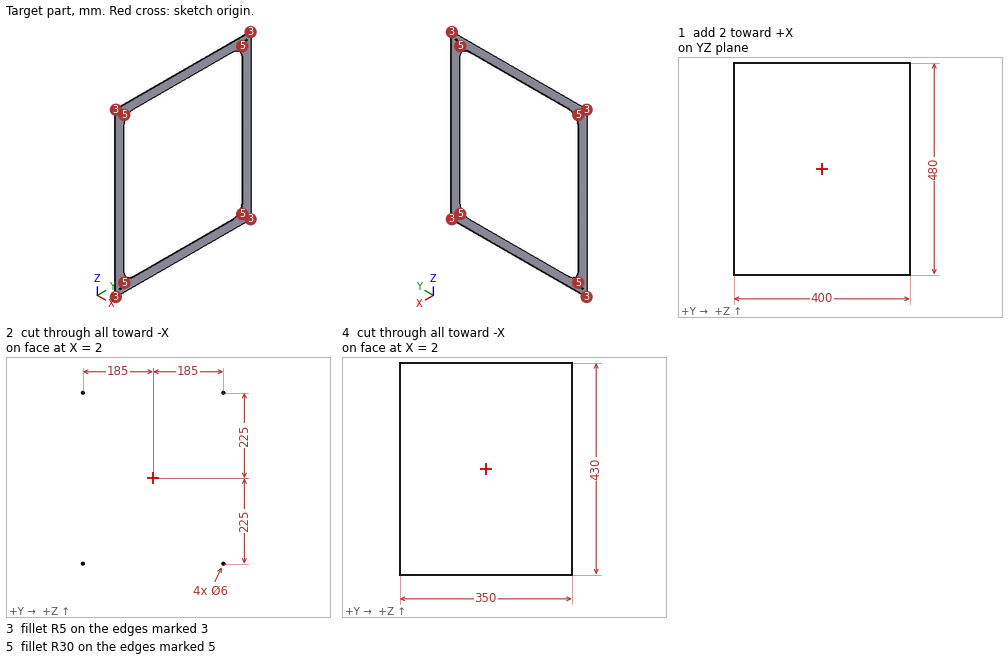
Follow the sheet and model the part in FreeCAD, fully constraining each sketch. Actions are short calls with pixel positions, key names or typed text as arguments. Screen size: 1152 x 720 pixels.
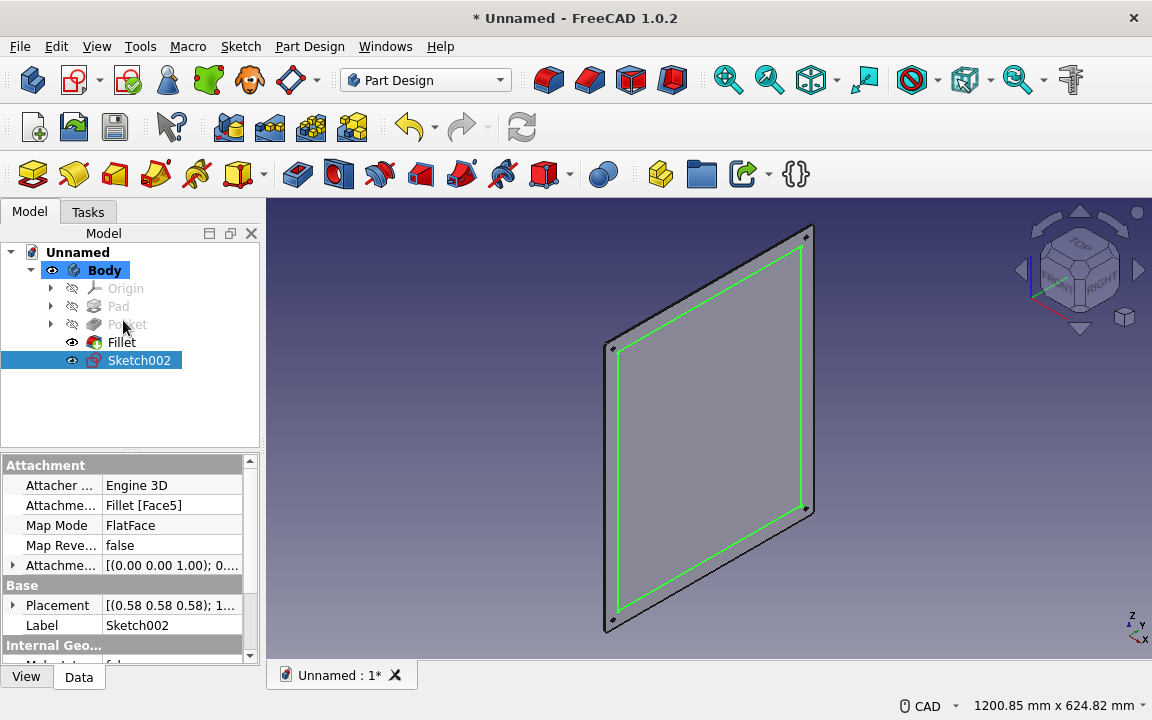
click(298, 174)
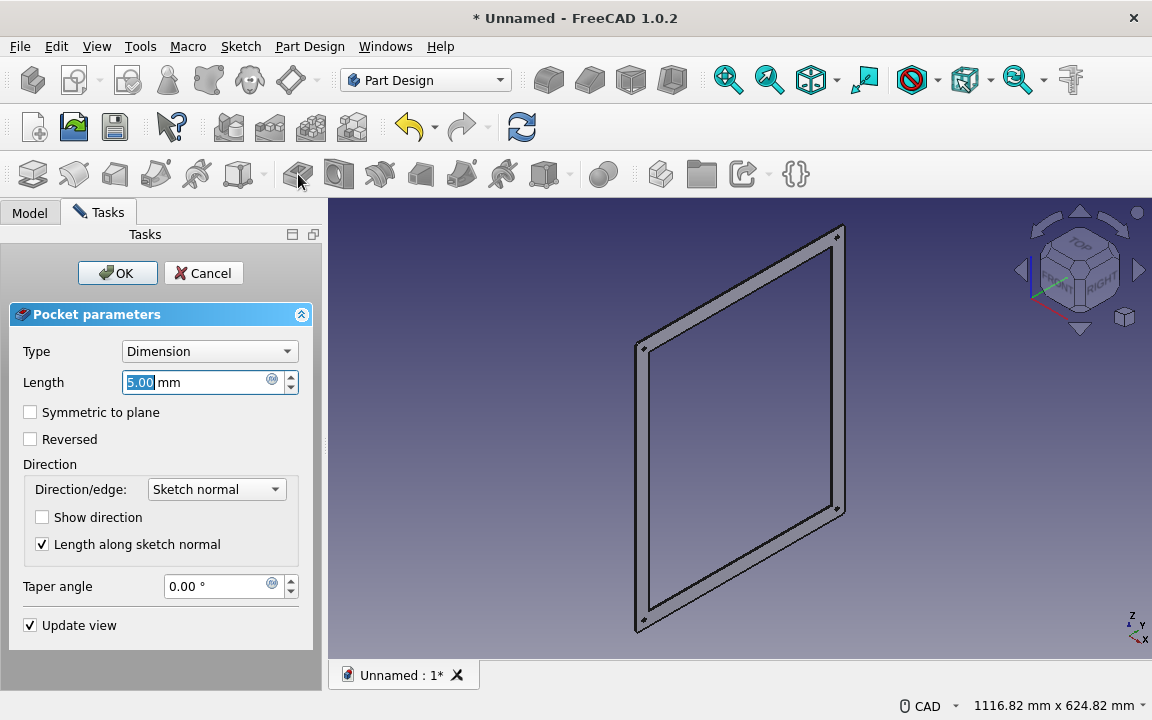
click(210, 352)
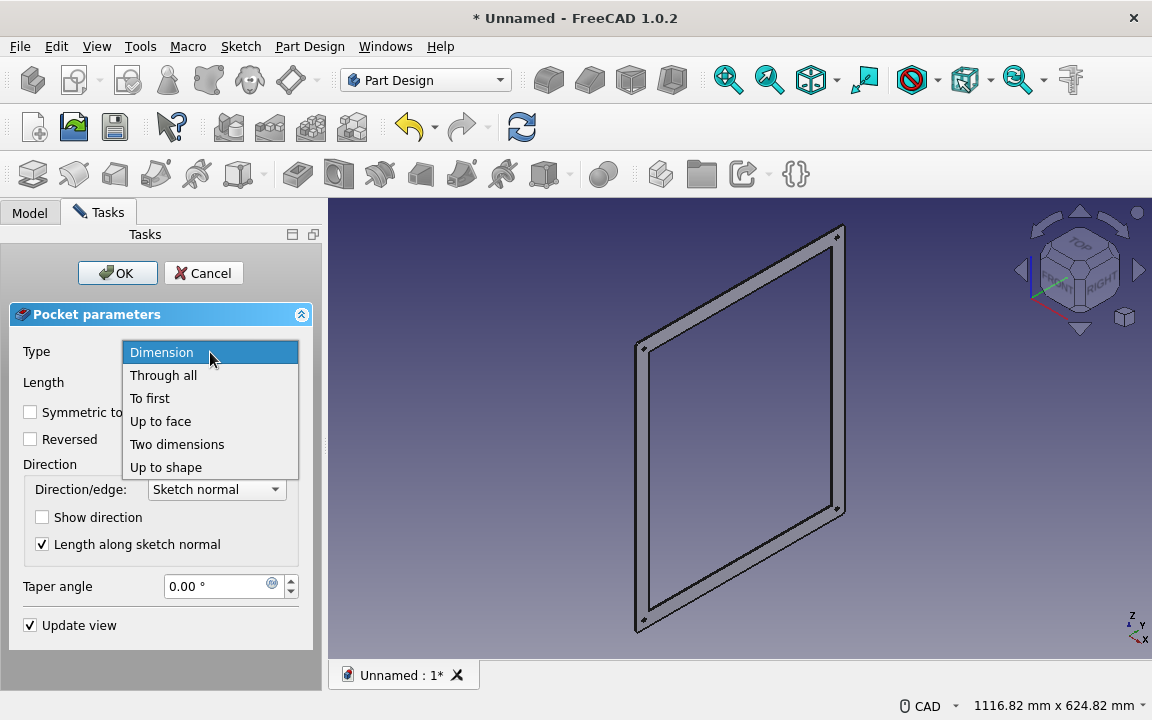
click(208, 376)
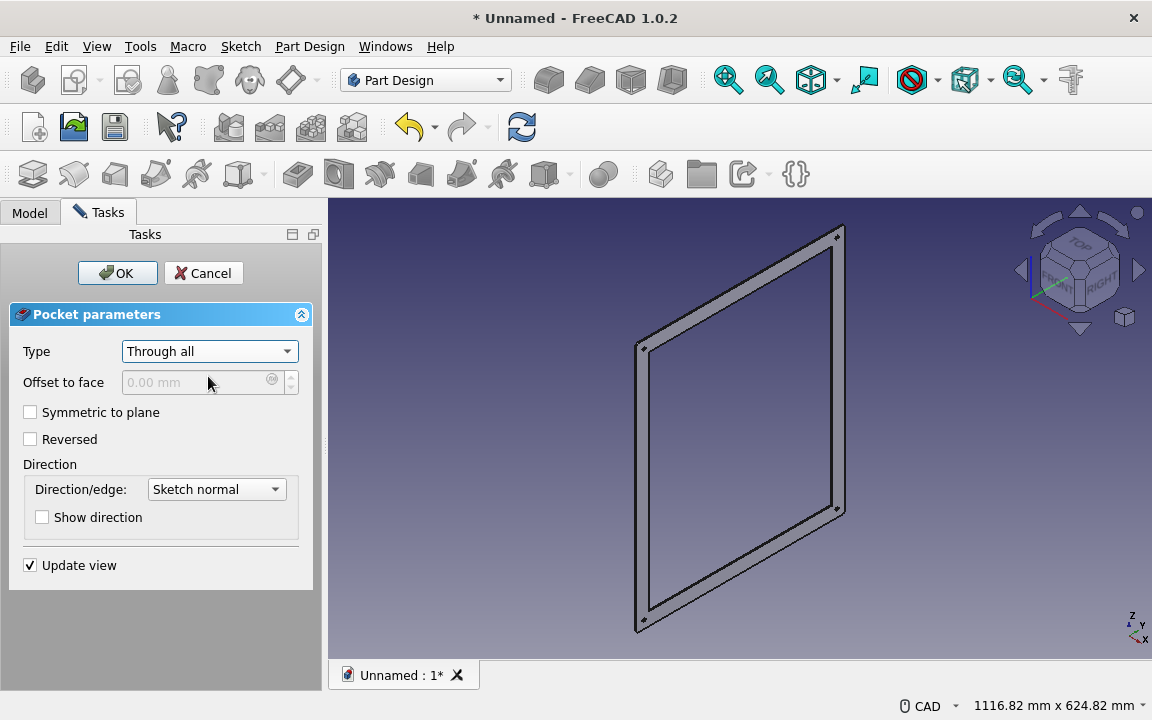
click(118, 273)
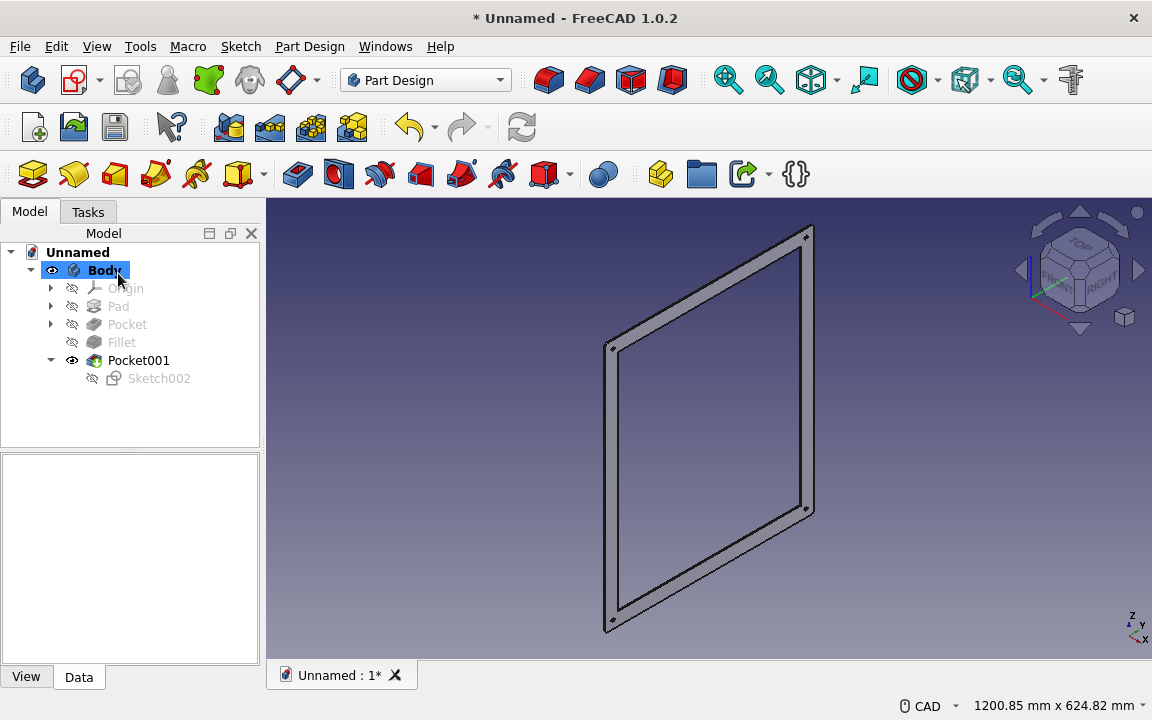
scroll(618, 351, up, 15)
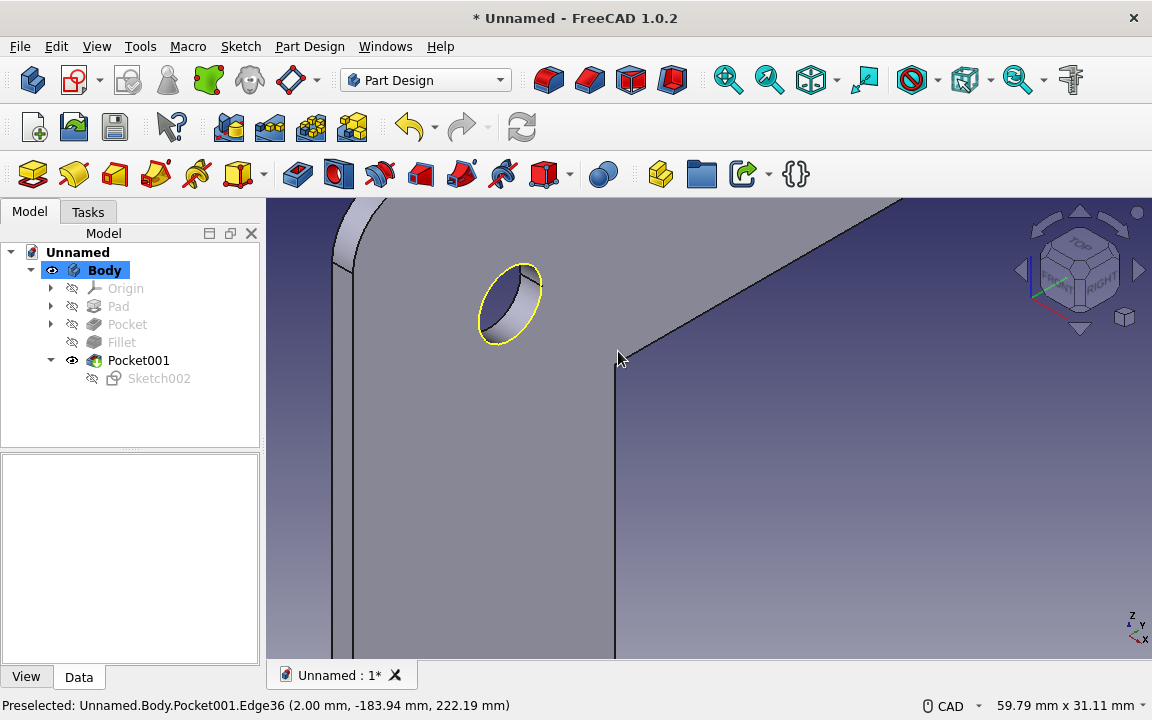
click(729, 80)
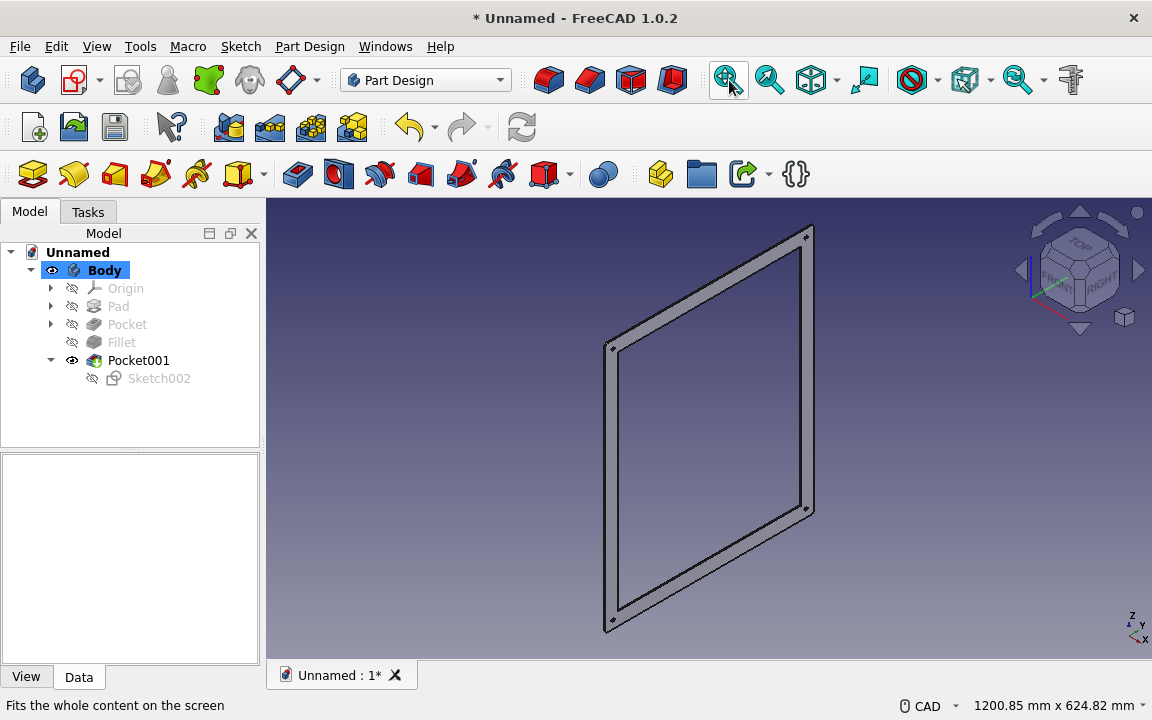
key(2)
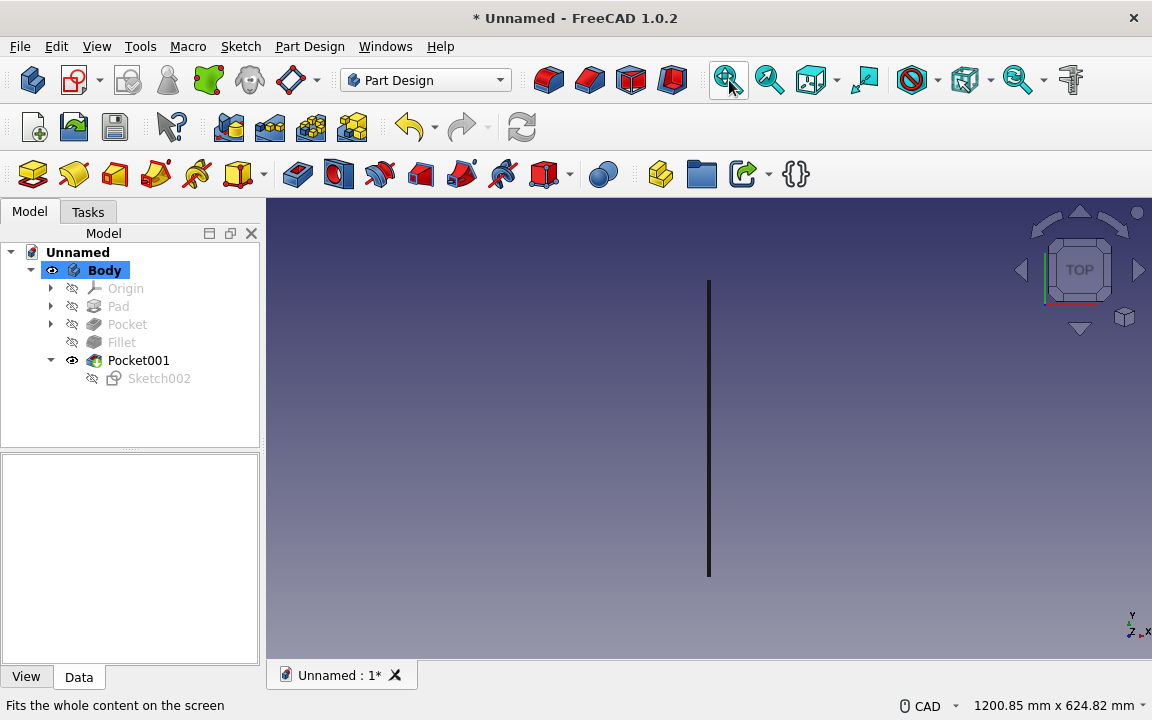
scroll(709, 557, up, 15)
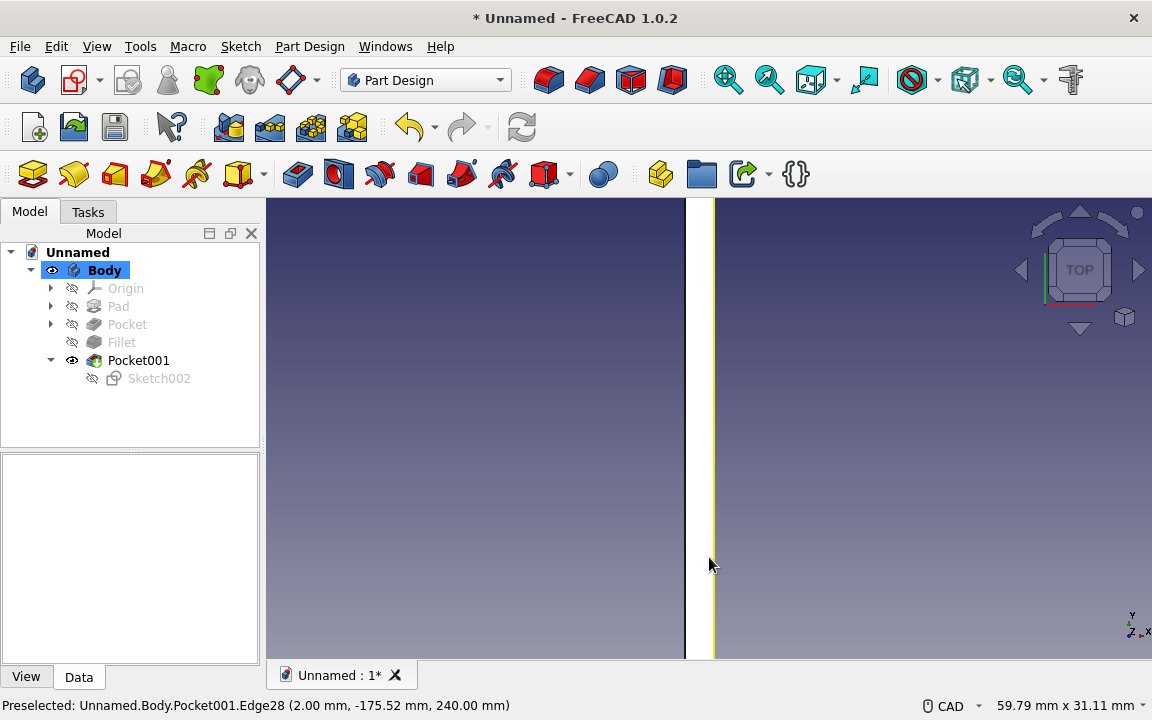
key(v)
key(f)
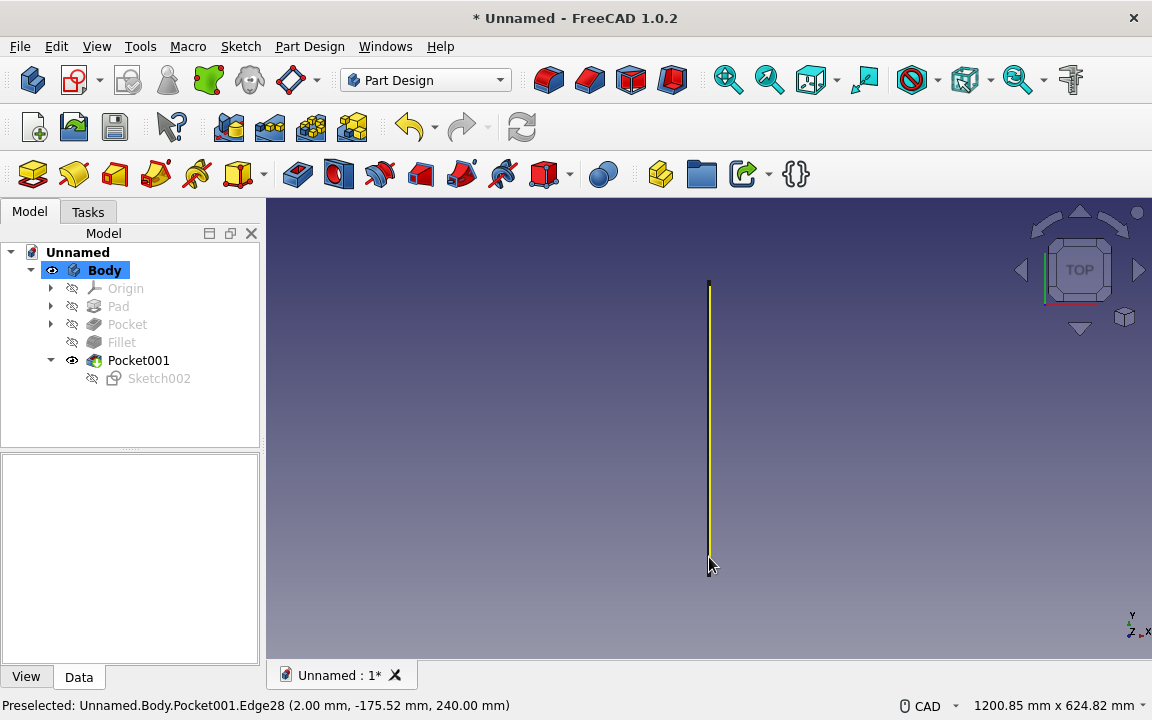
key(0)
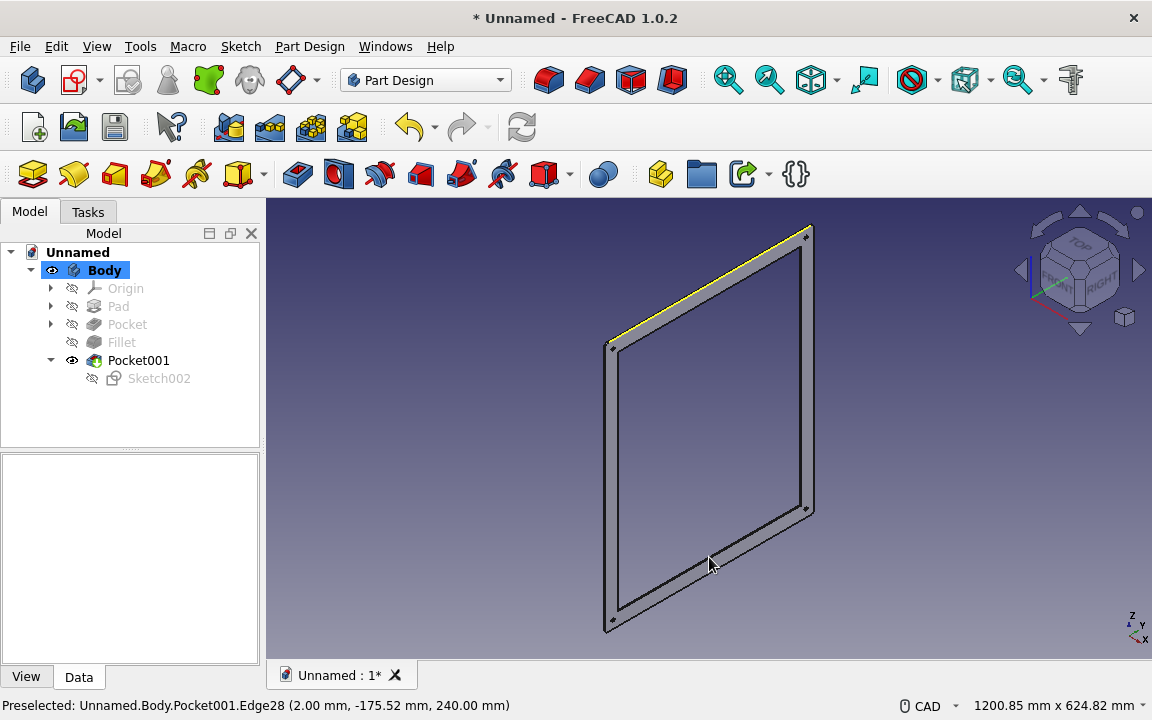
scroll(618, 351, up, 15)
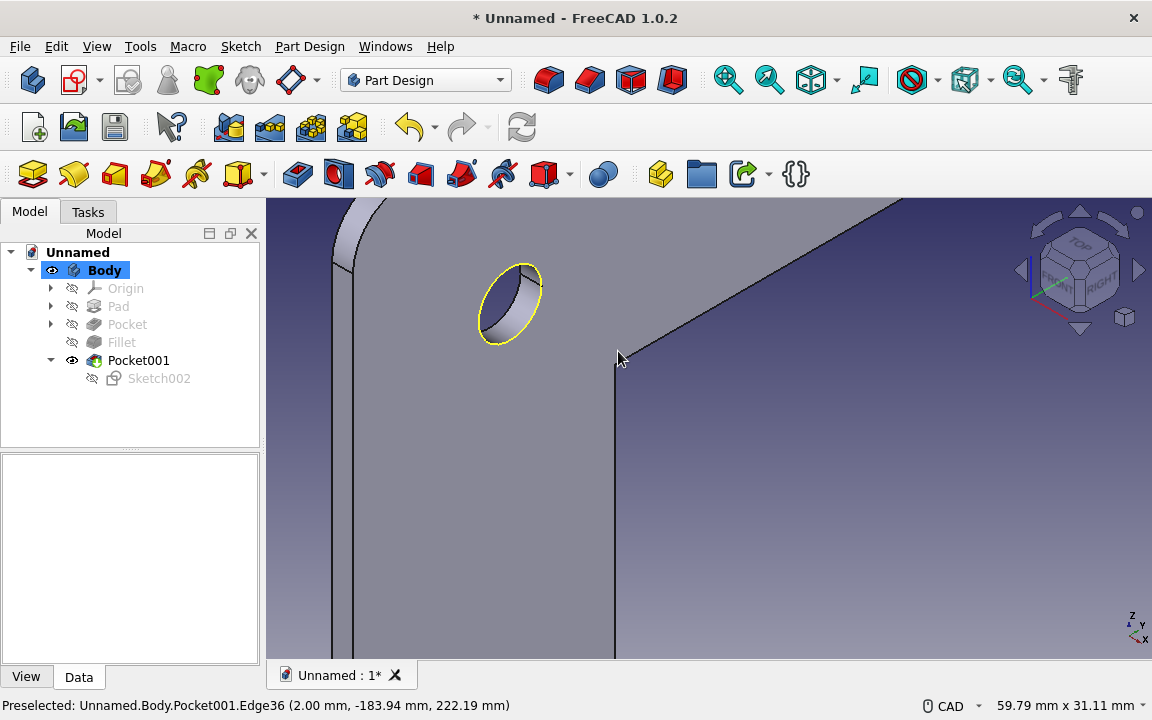
click(729, 80)